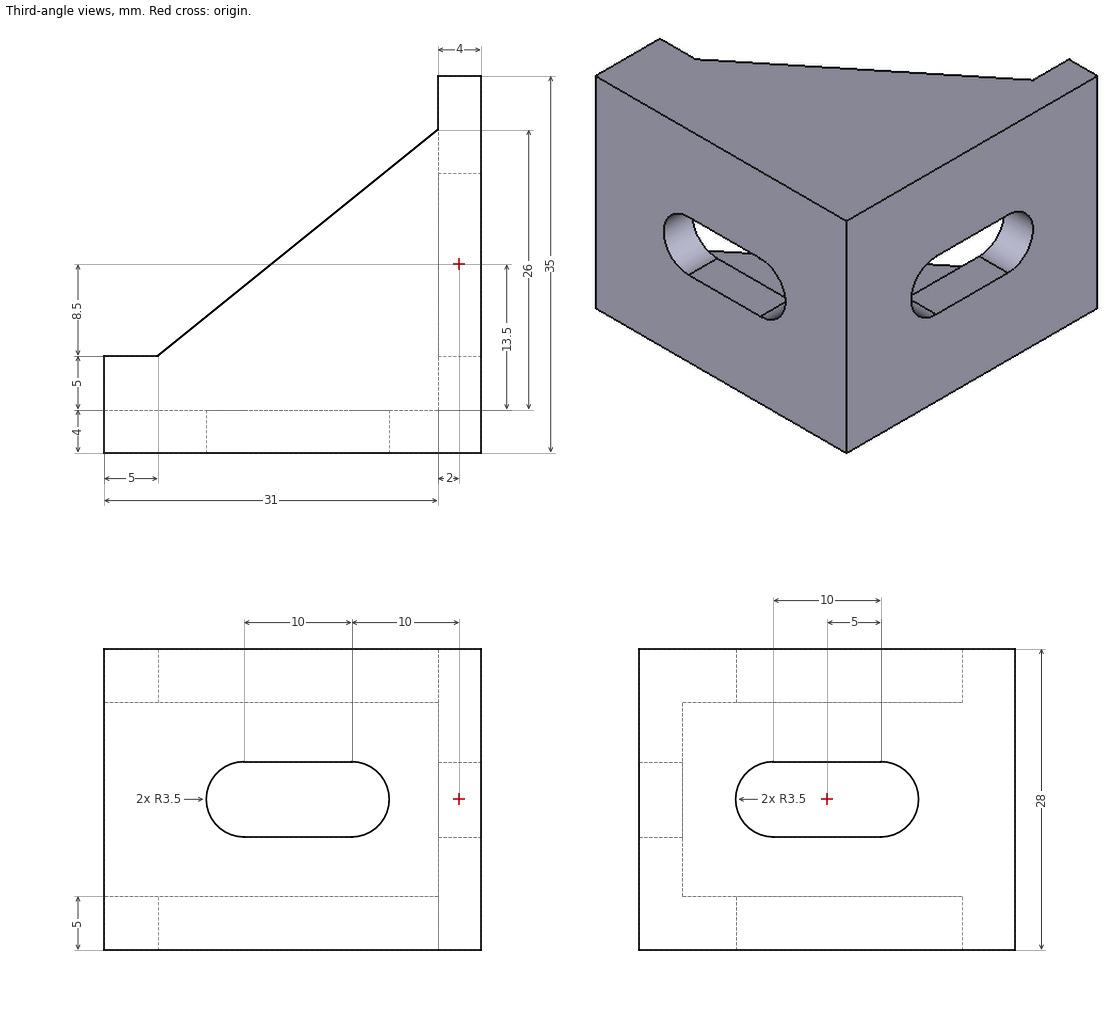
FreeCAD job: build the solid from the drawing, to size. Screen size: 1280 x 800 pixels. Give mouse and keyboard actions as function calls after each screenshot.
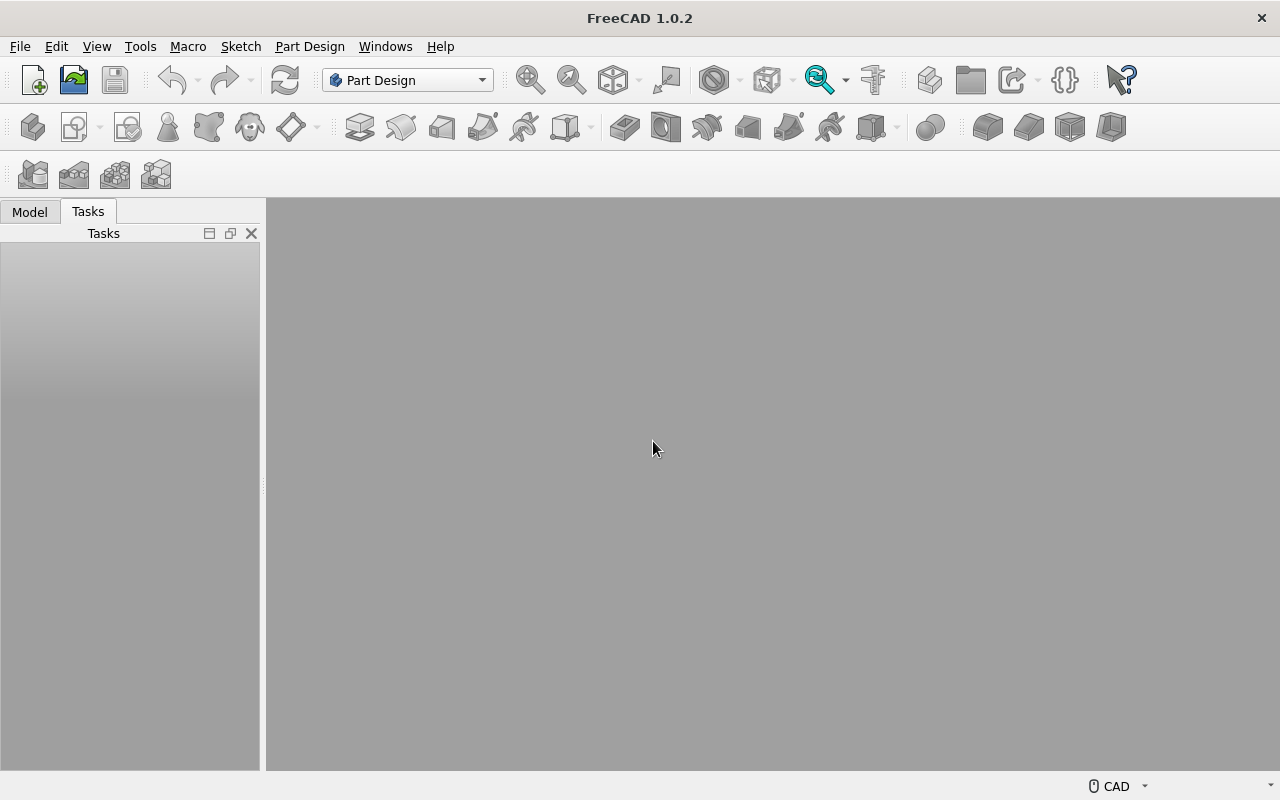
click(33, 80)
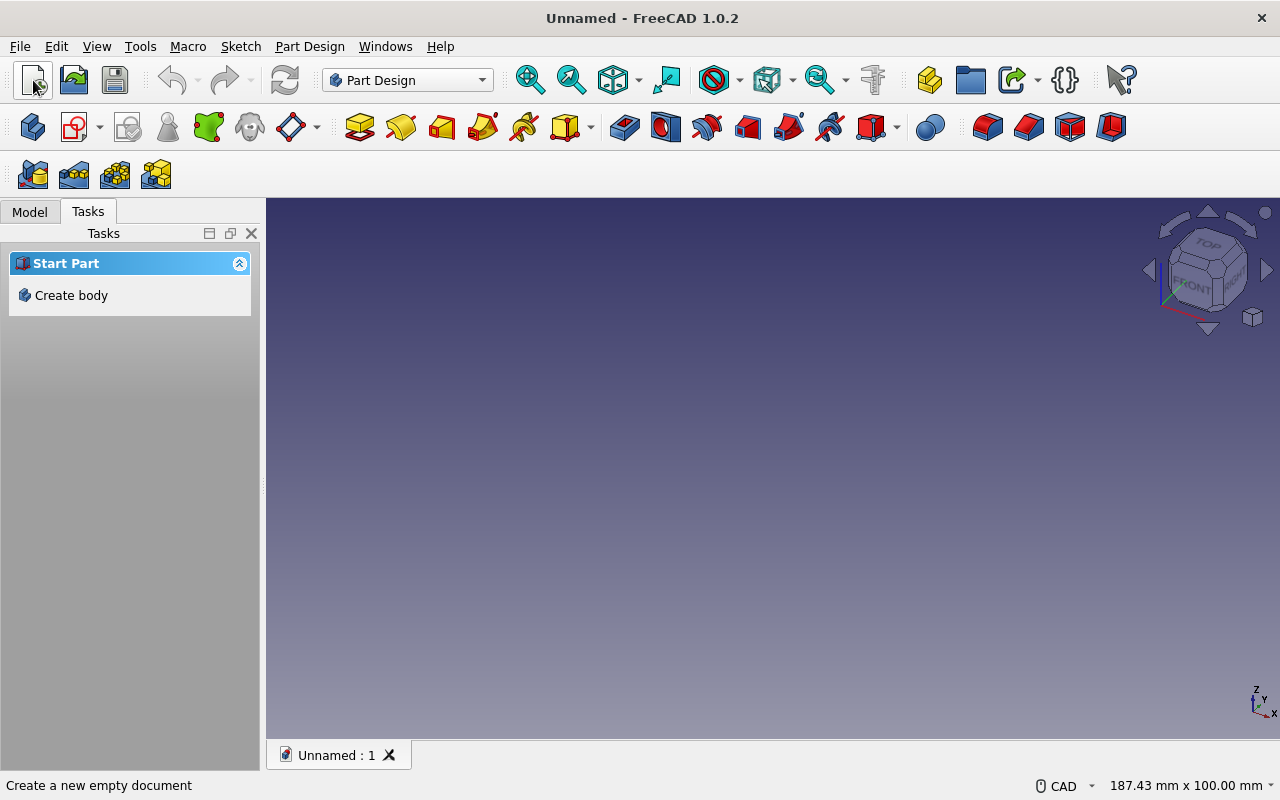
click(74, 128)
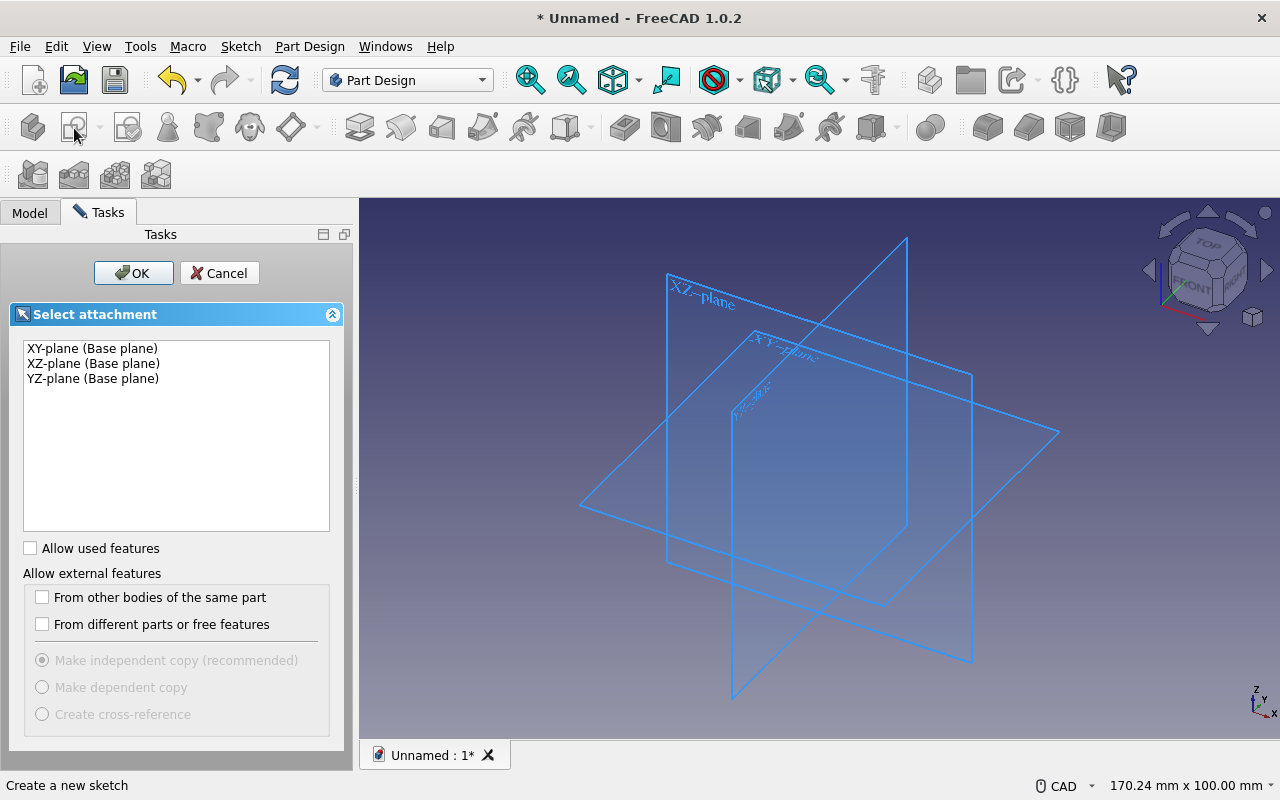
click(84, 348)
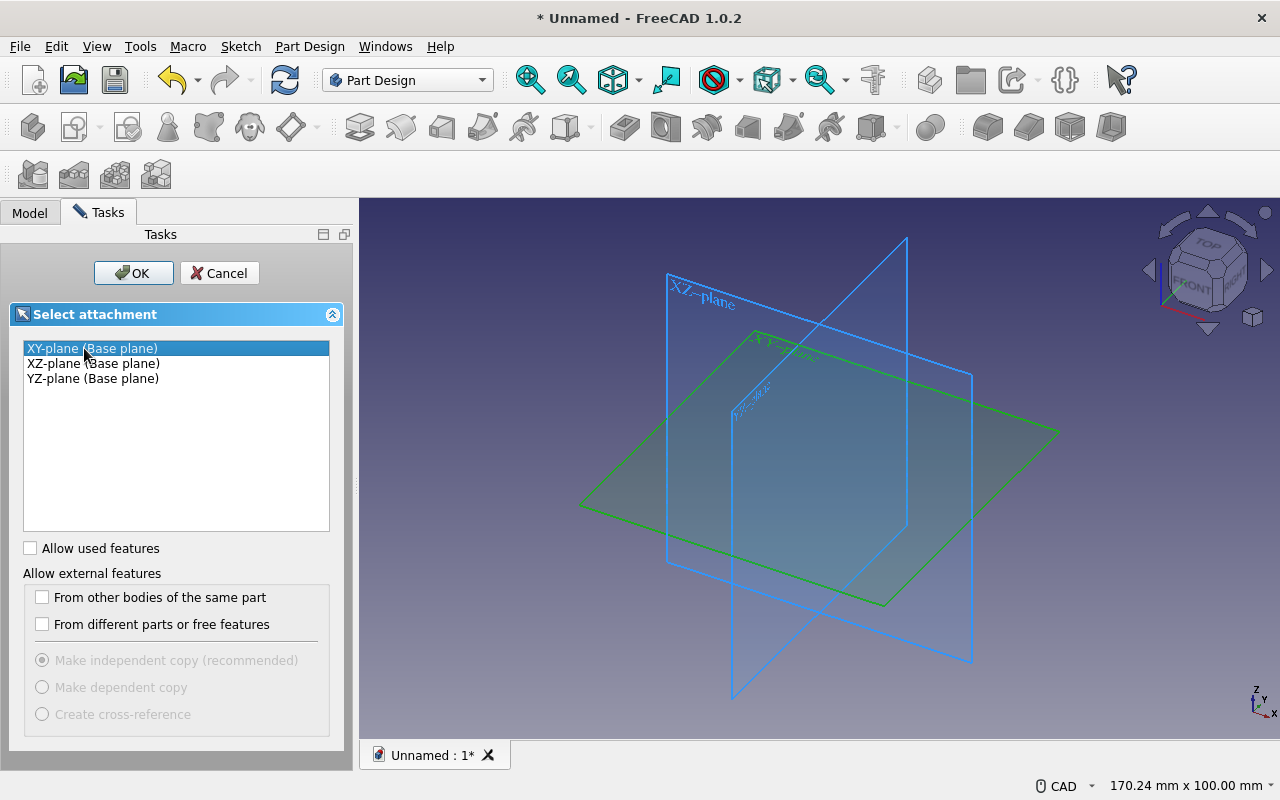
click(134, 273)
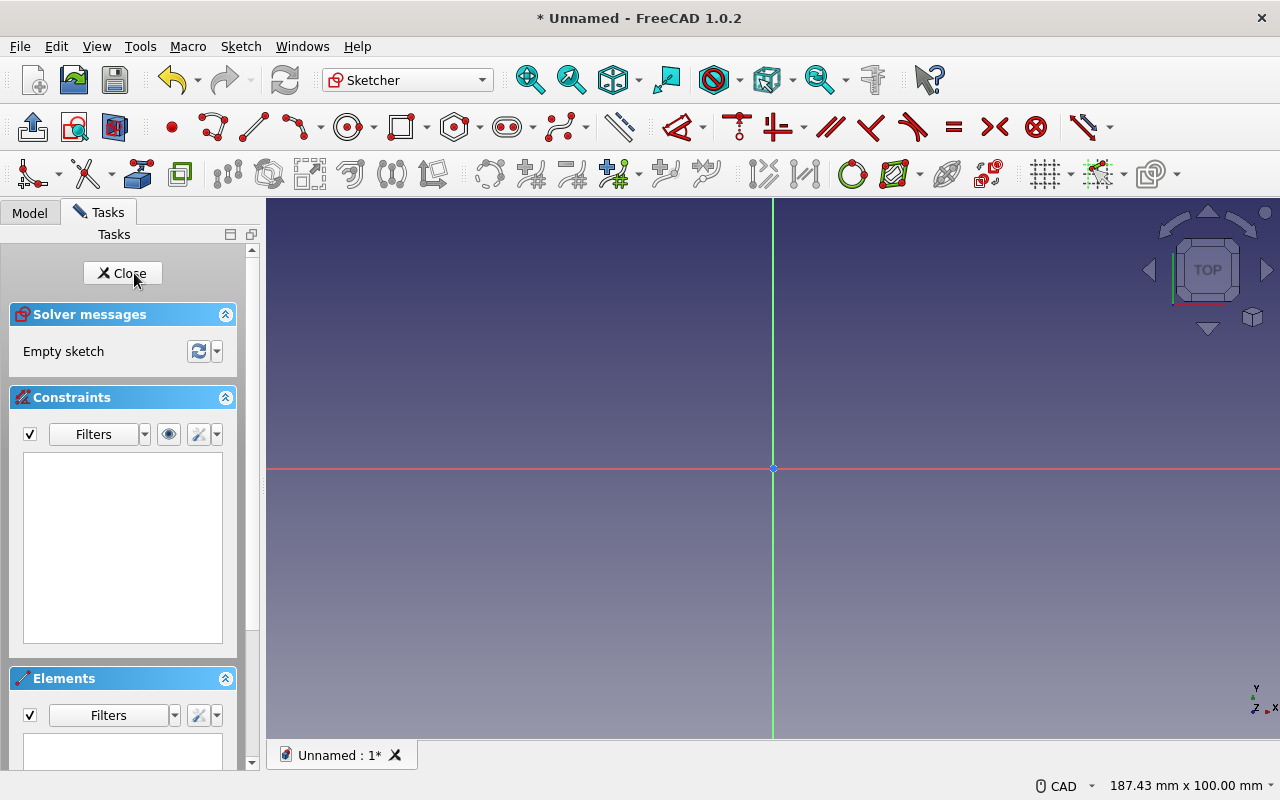
scroll(670, 468, up, 3)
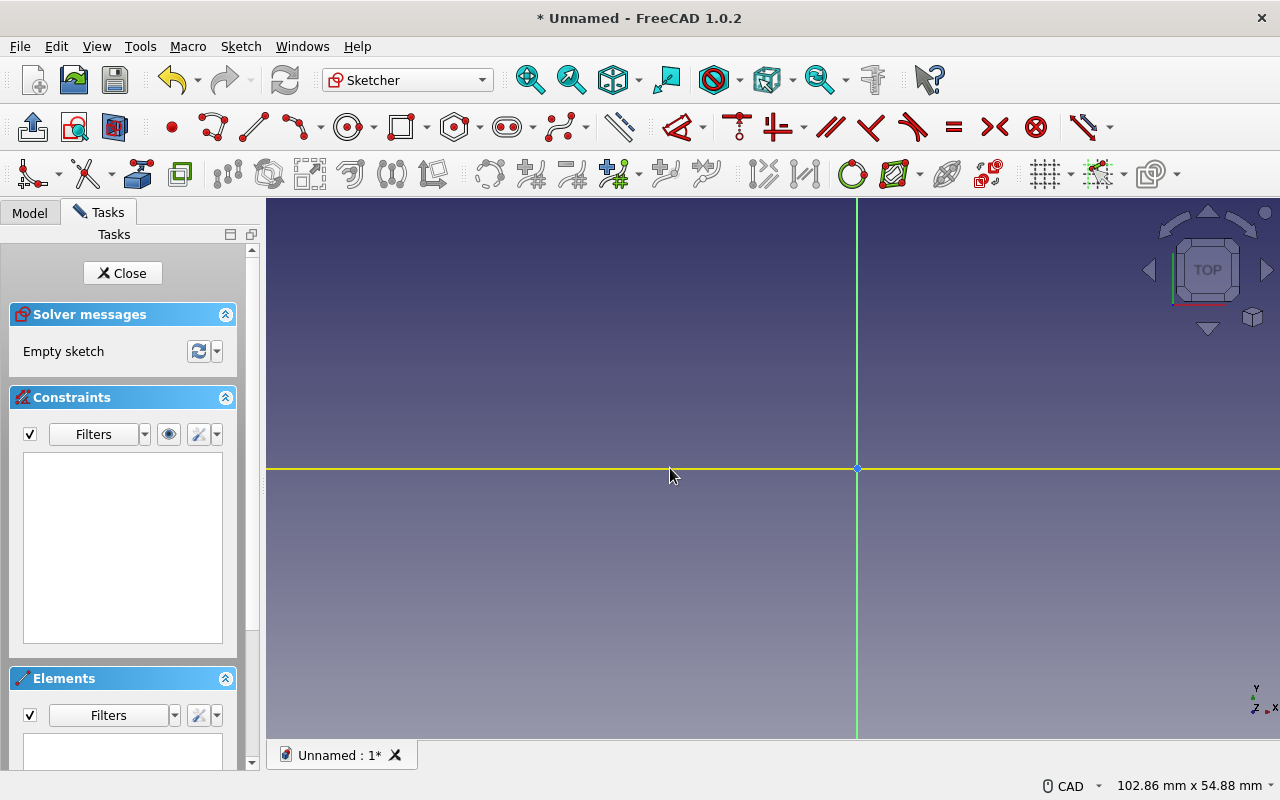
click(213, 128)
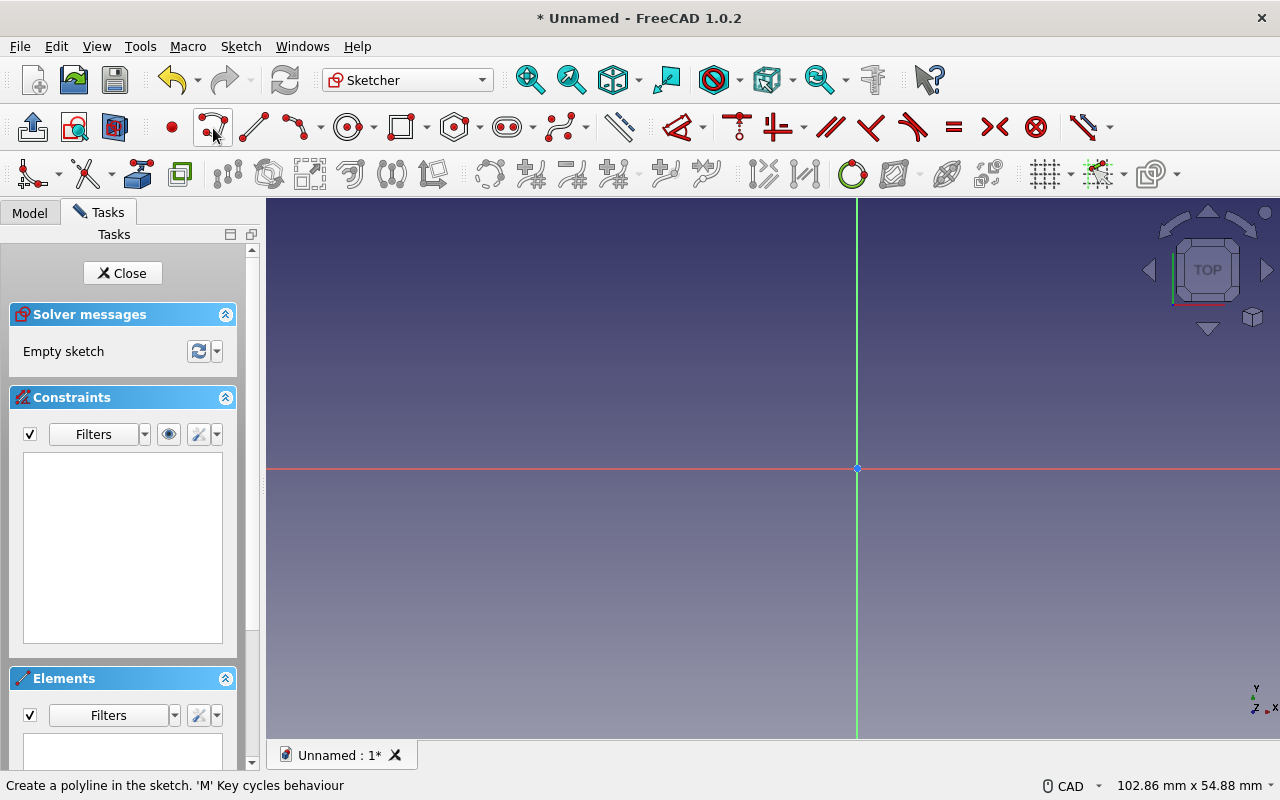
click(838, 602)
click(532, 602)
click(532, 641)
click(877, 641)
click(877, 296)
click(838, 296)
click(838, 603)
key(Escape)
key(Escape)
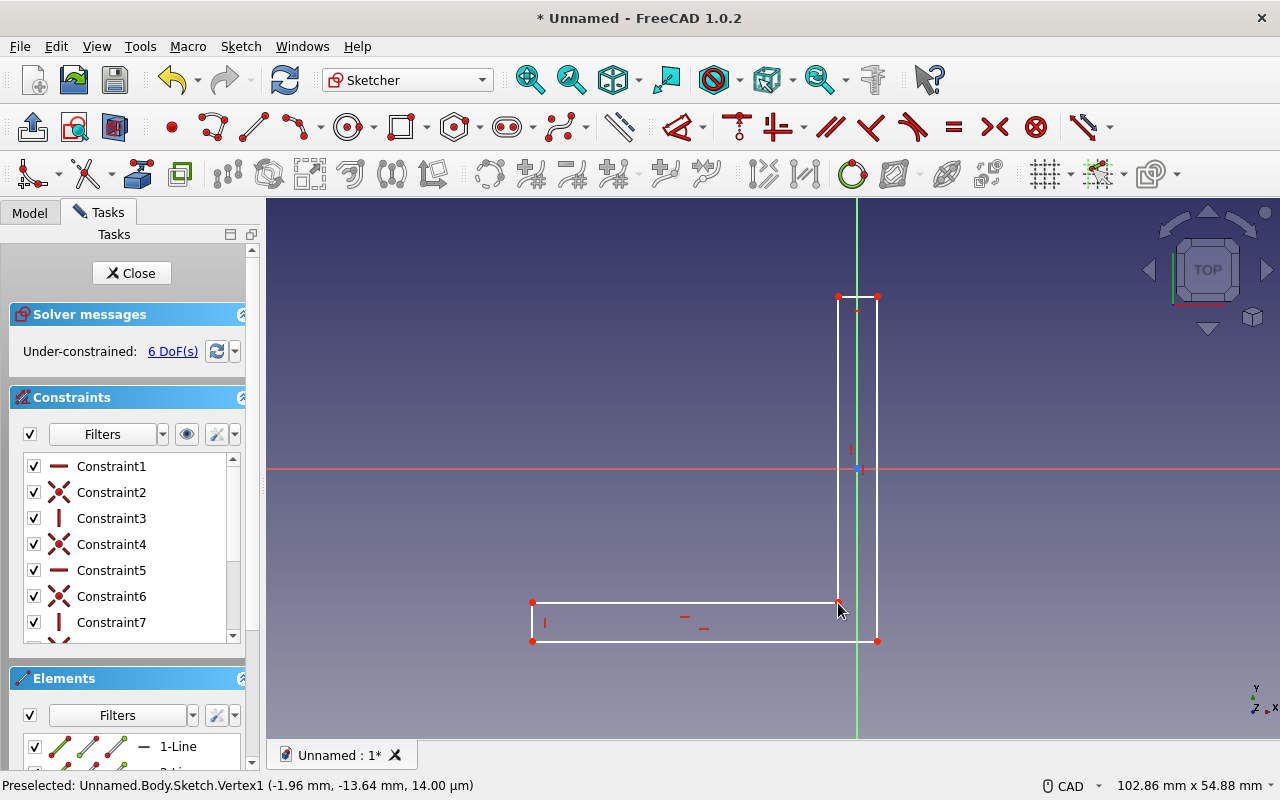
click(532, 615)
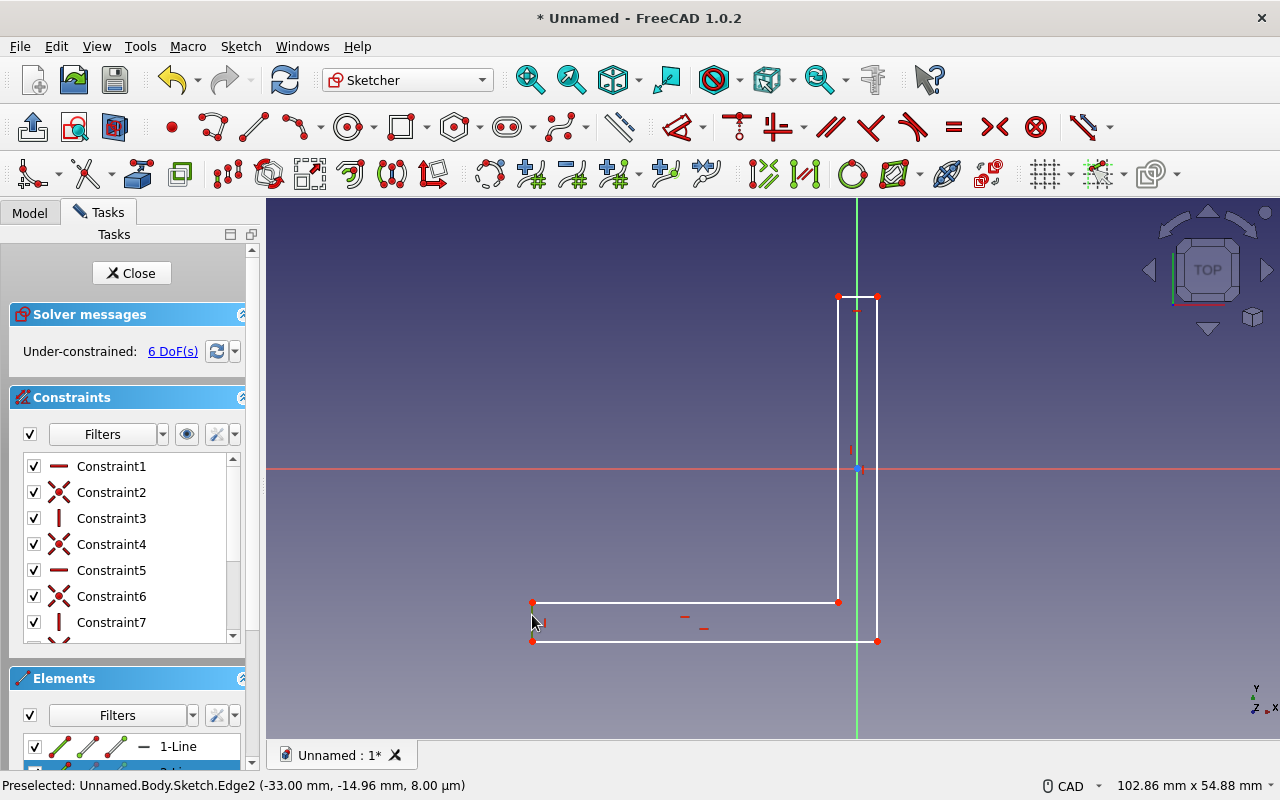
click(702, 128)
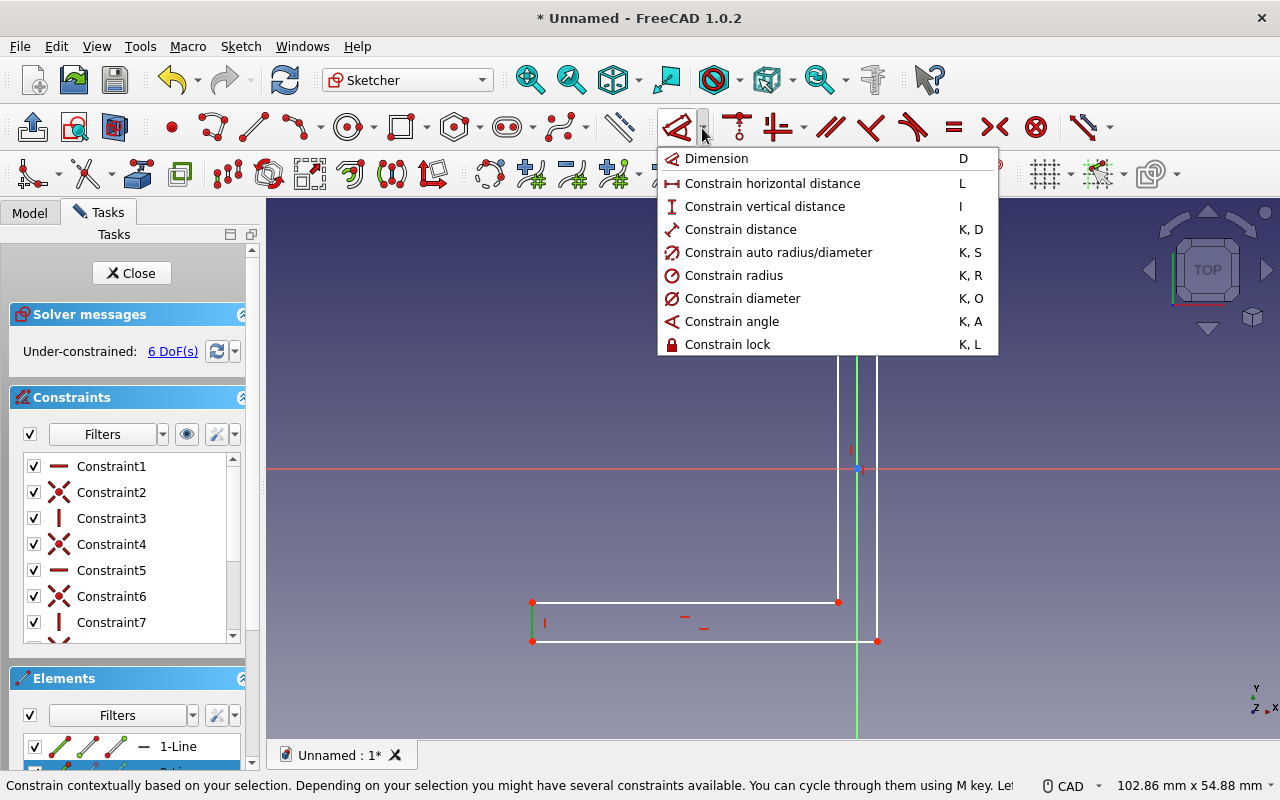
click(828, 206)